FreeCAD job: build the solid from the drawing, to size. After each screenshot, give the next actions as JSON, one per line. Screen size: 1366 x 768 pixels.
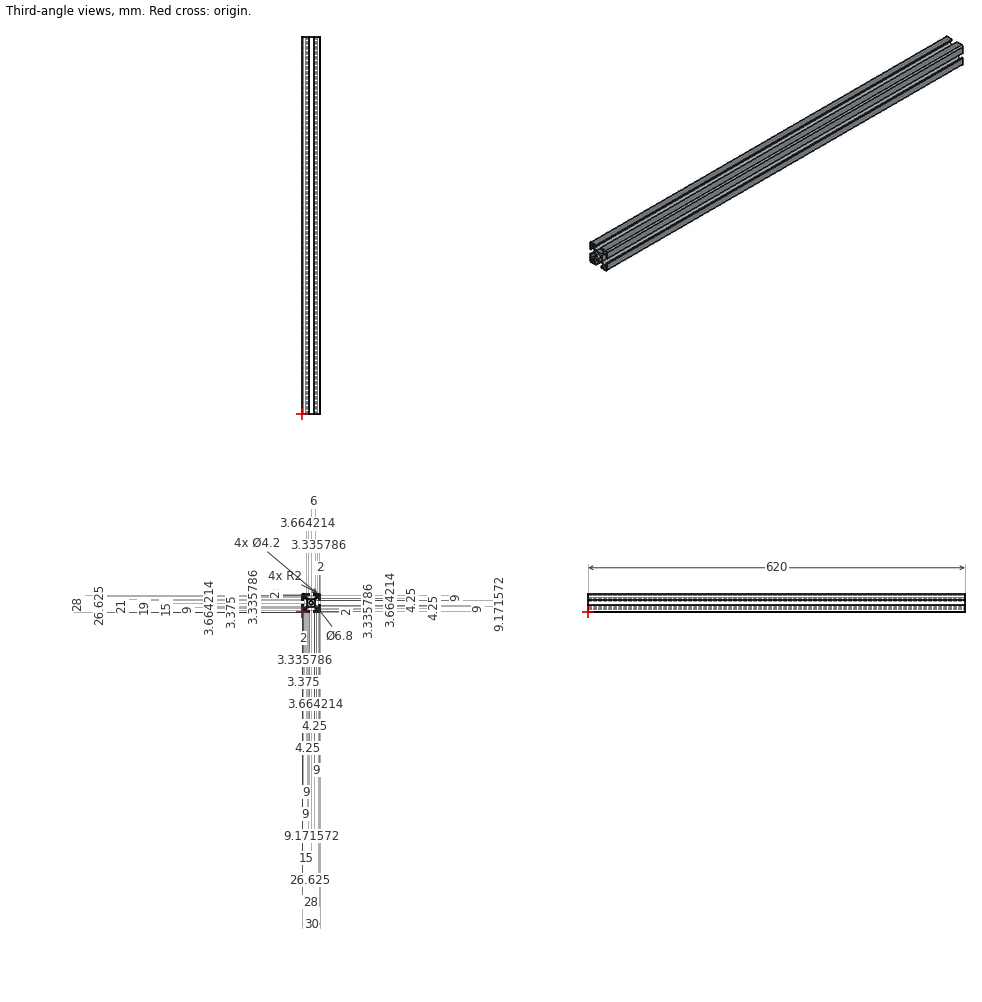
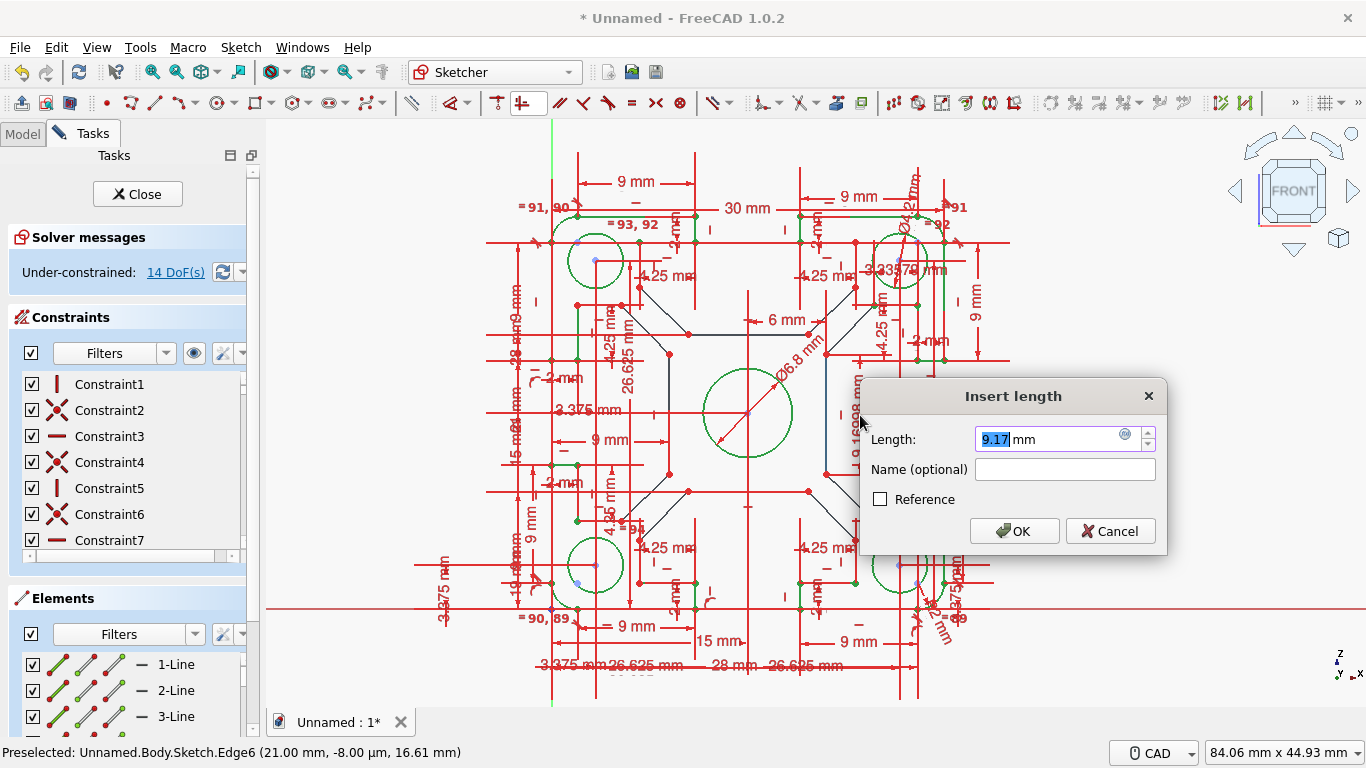
{"action": "type", "text": "9.171572"}
{"action": "key", "text": "Return"}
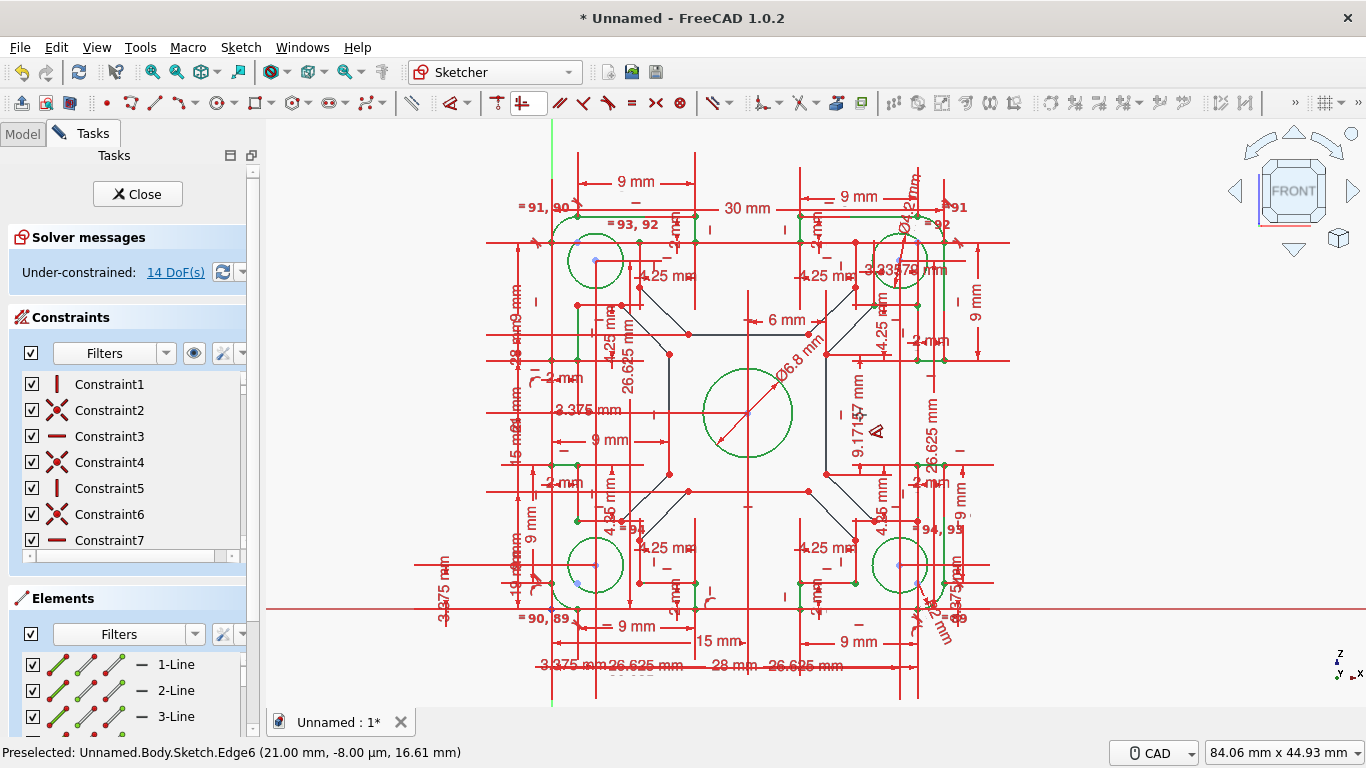
{"action": "left_click", "coordinate": [887, 521]}
{"action": "left_click", "coordinate": [906, 555]}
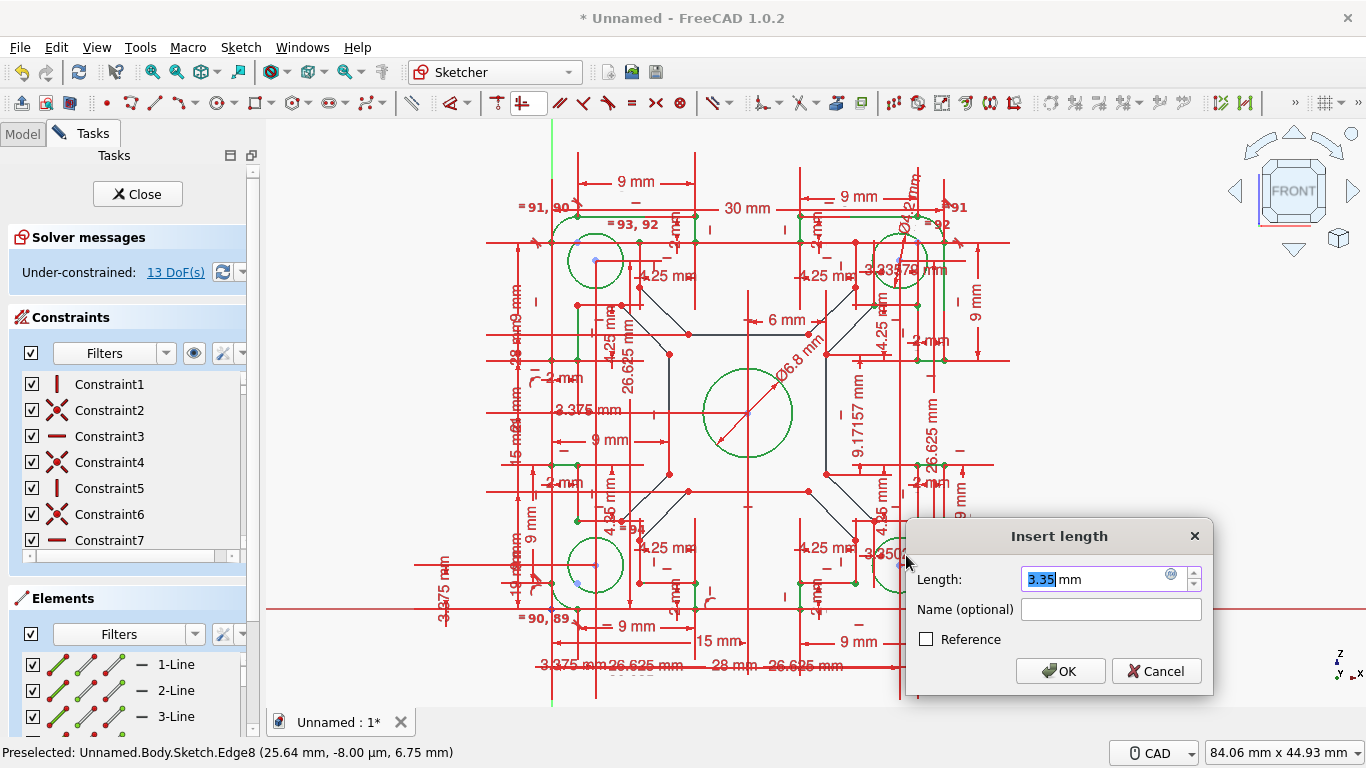
{"action": "type", "text": "3.335786"}
{"action": "key", "text": "Return"}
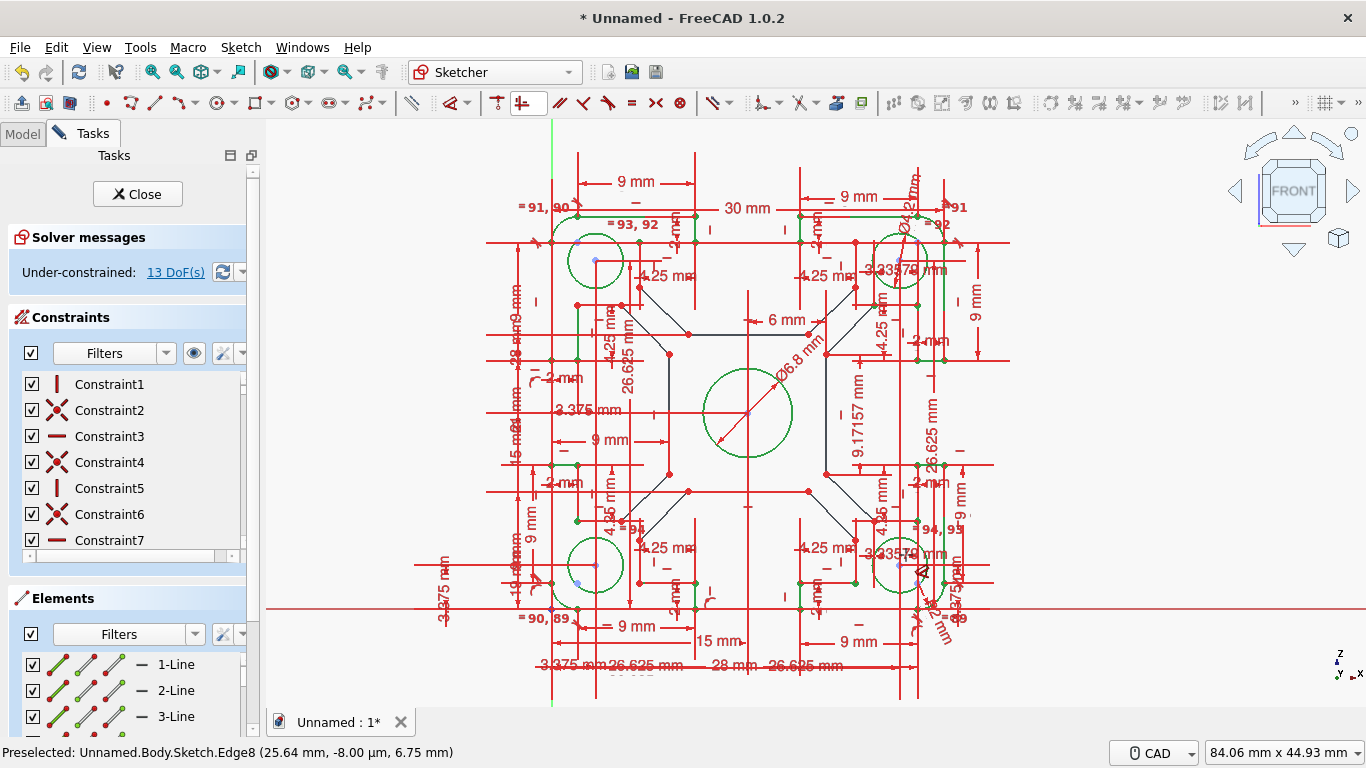
{"action": "left_click", "coordinate": [856, 570]}
{"action": "left_click", "coordinate": [774, 572]}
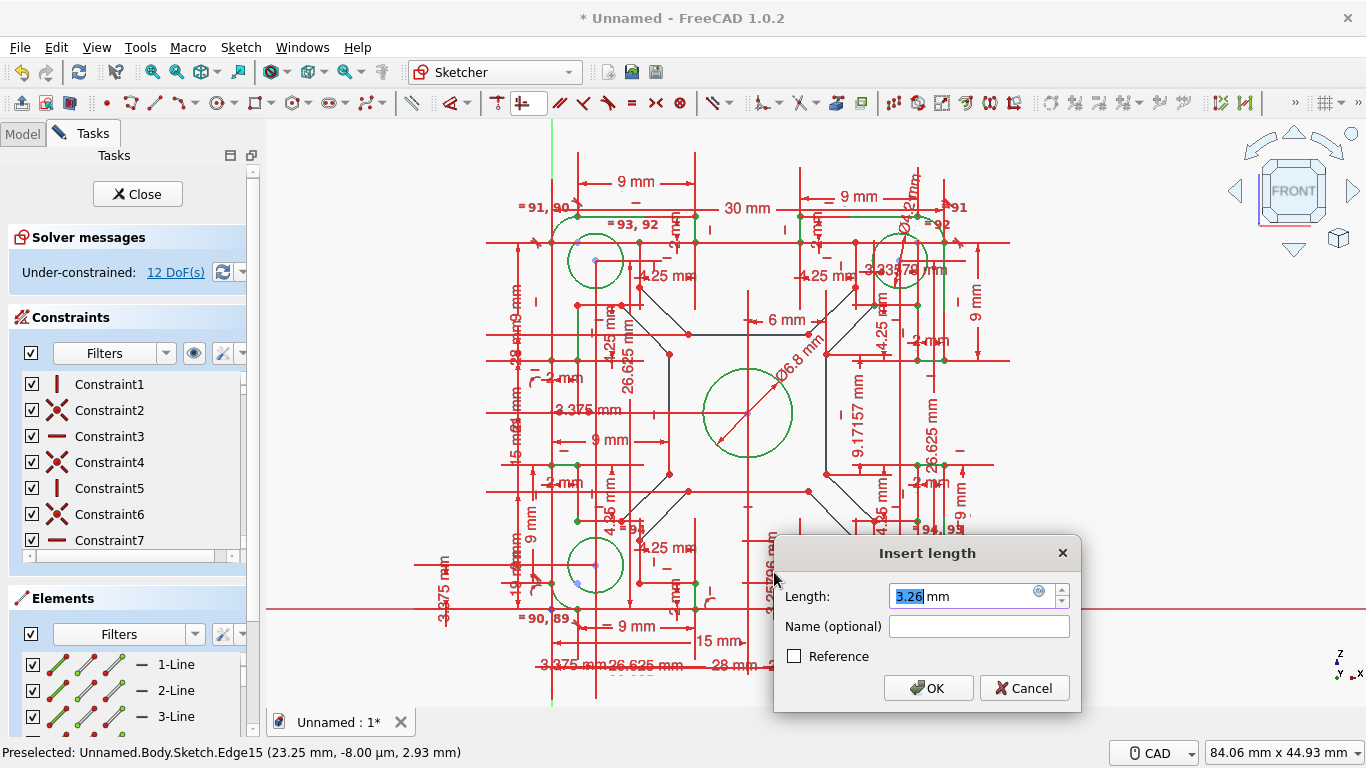
{"action": "type", "text": "3.335786"}
{"action": "key", "text": "Return"}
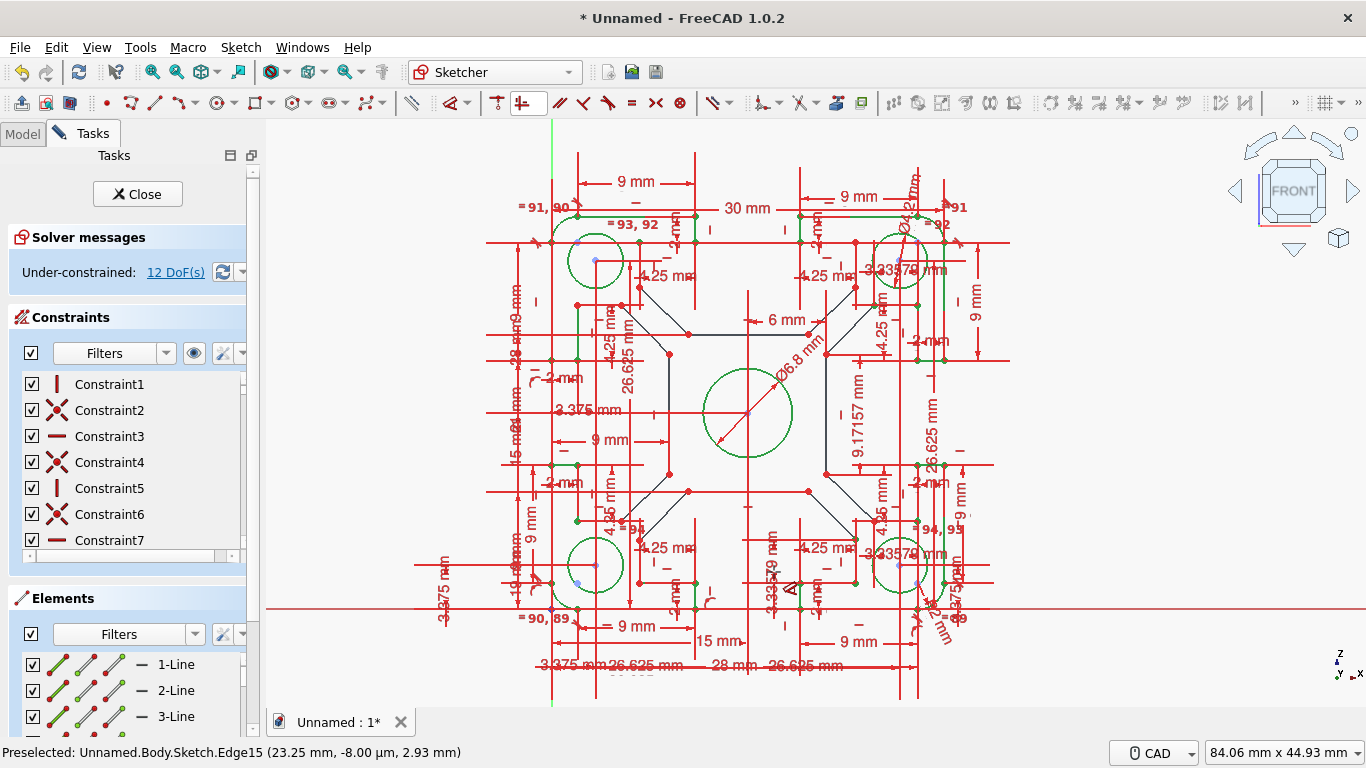
{"action": "left_click", "coordinate": [772, 492]}
{"action": "left_click", "coordinate": [748, 526]}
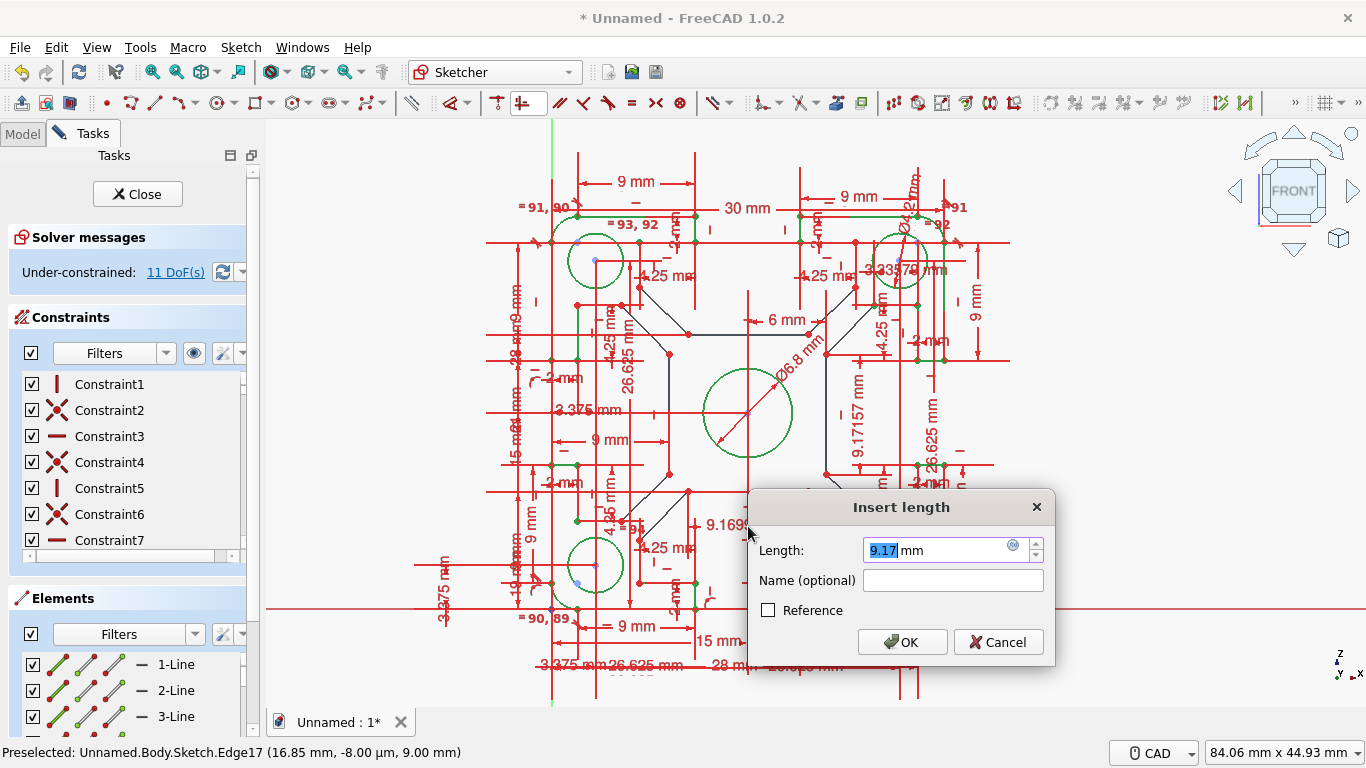
{"action": "type", "text": "9.171572"}
{"action": "key", "text": "Return"}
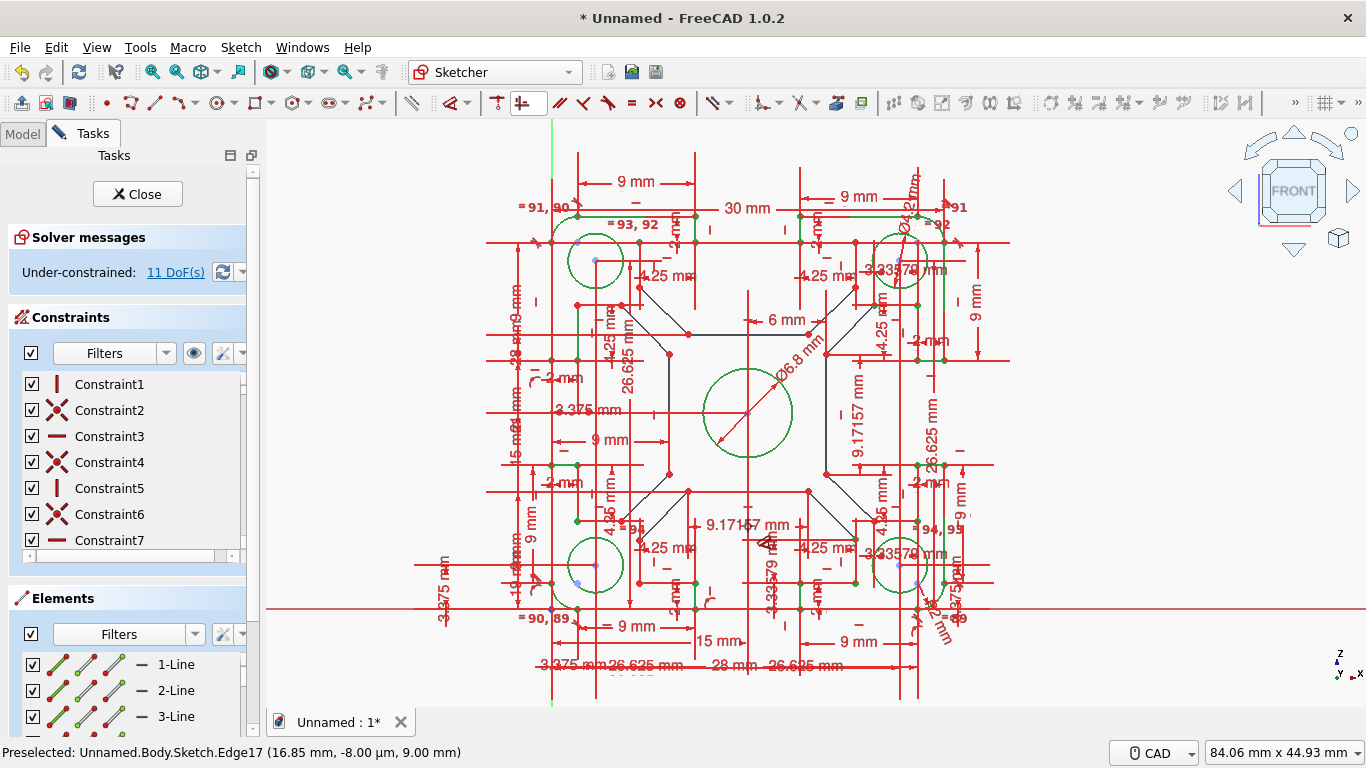
{"action": "left_click", "coordinate": [640, 553]}
{"action": "left_click", "coordinate": [606, 572]}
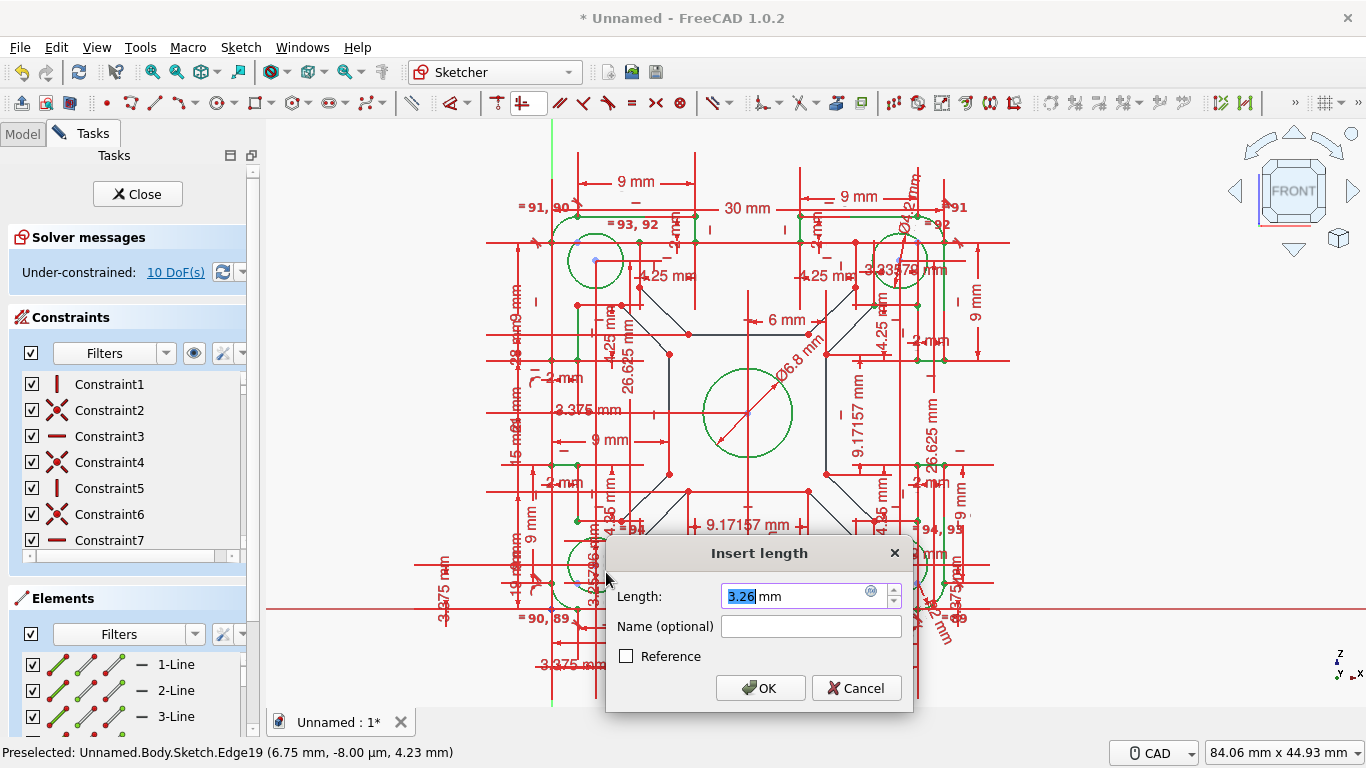
{"action": "type", "text": "3.335786"}
{"action": "key", "text": "Return"}